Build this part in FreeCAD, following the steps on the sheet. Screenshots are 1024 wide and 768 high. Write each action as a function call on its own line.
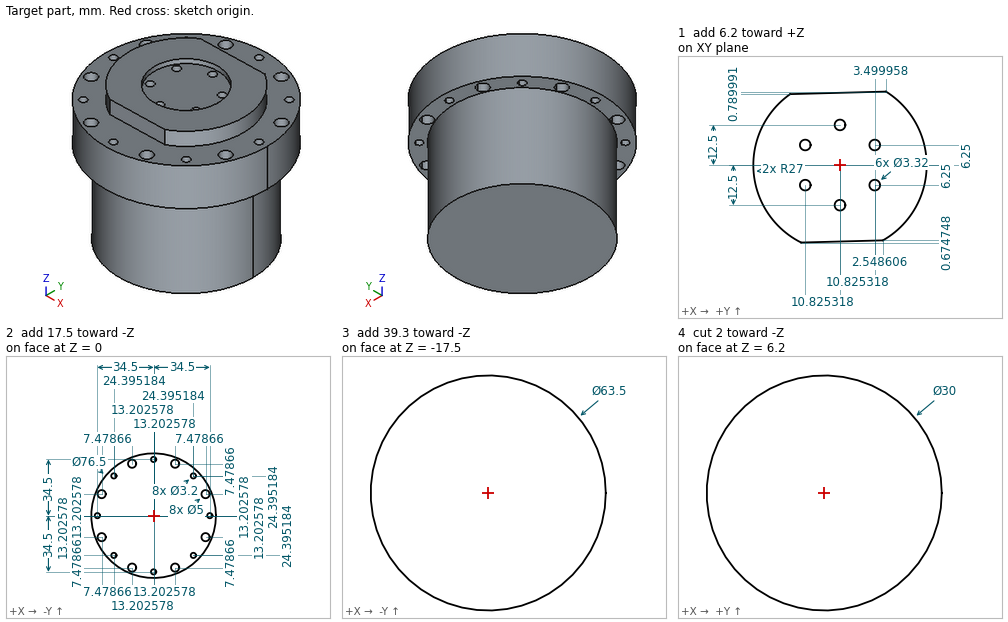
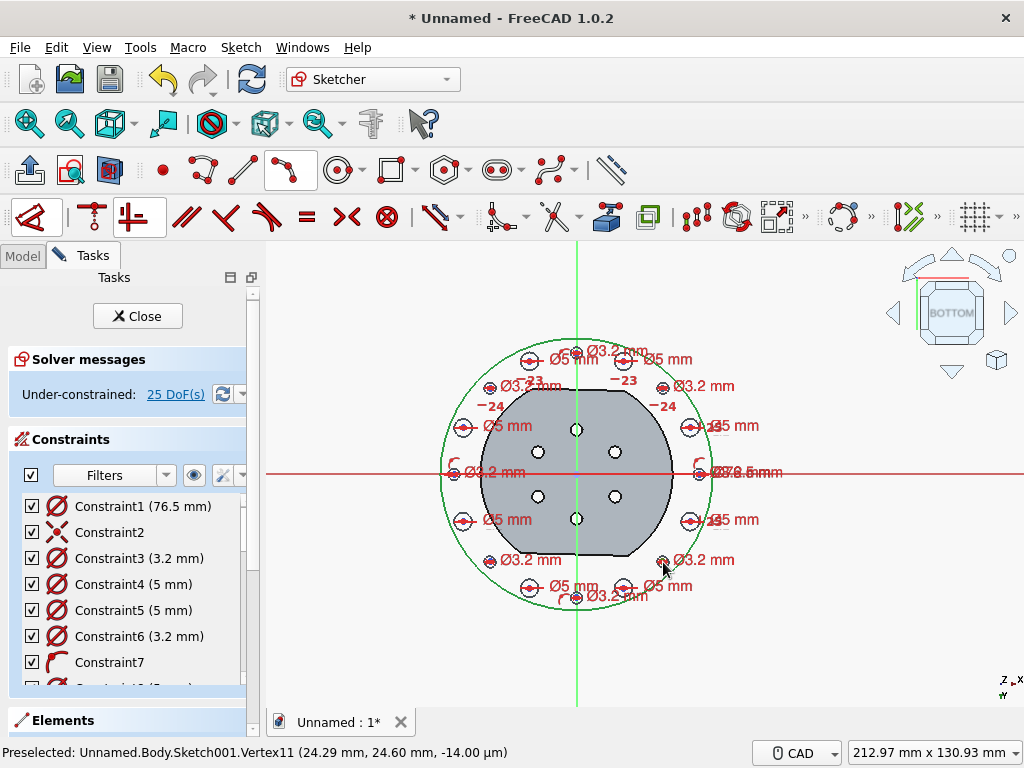
click(160, 218)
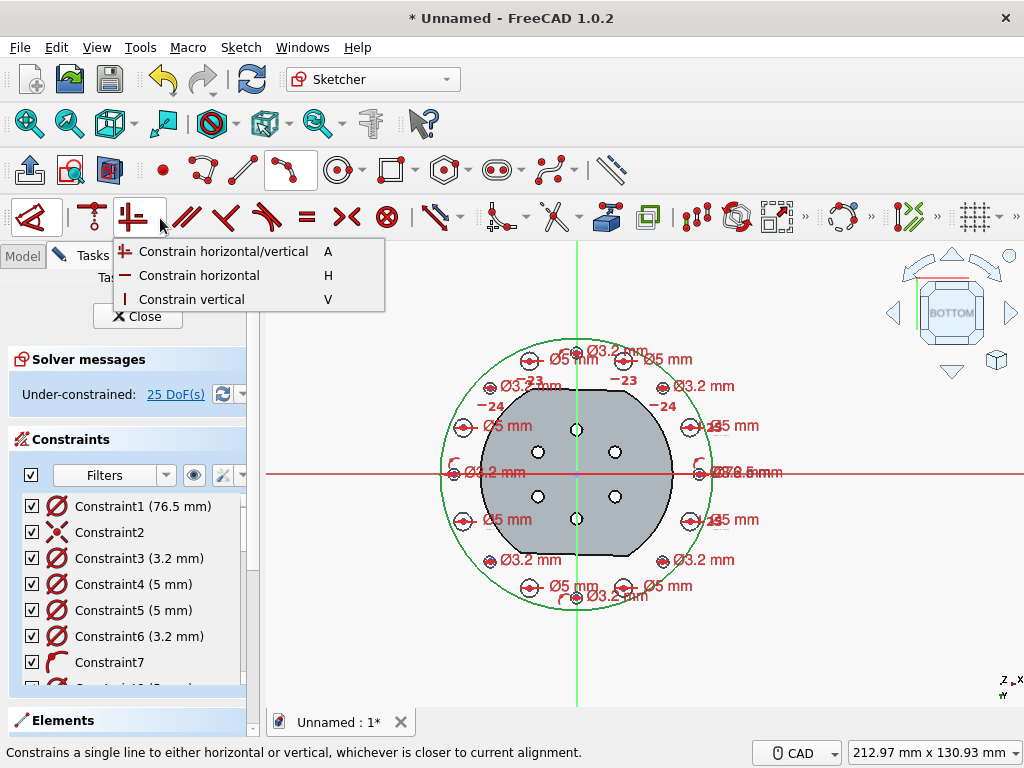
click(249, 299)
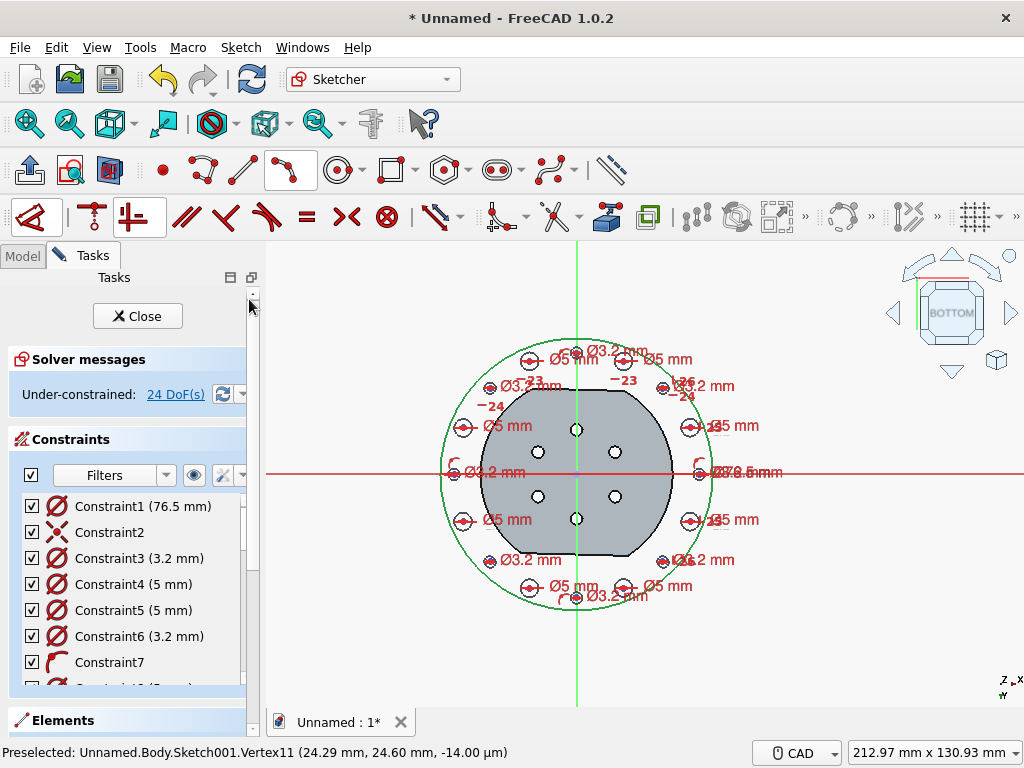
click(463, 428)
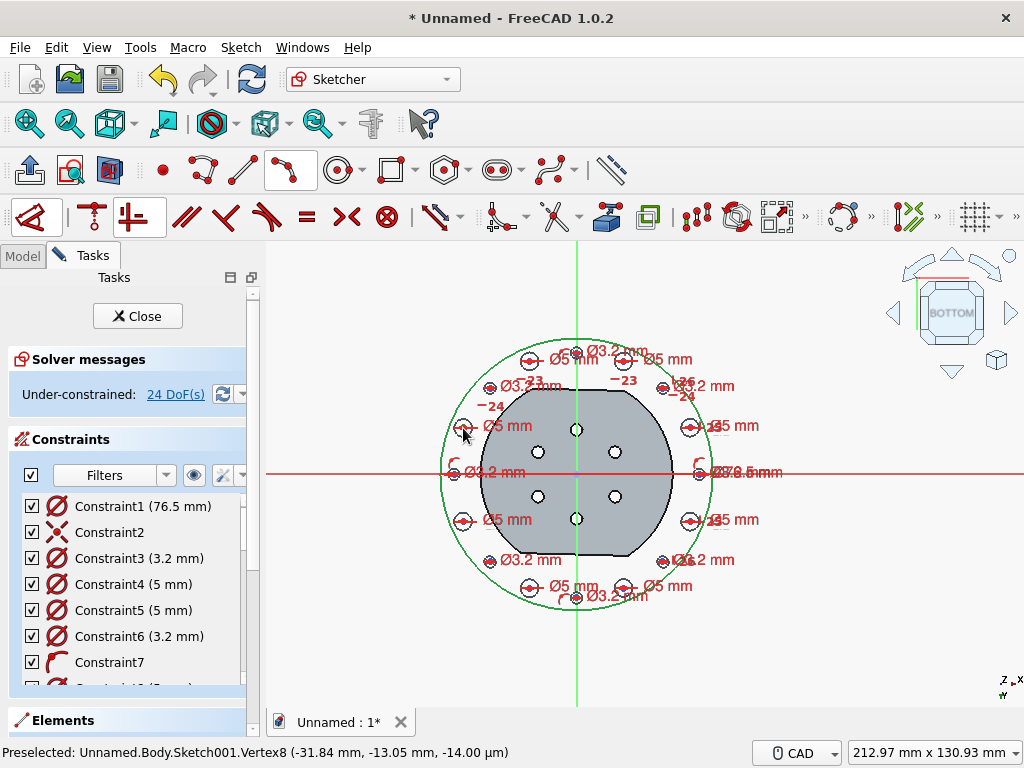
click(463, 522)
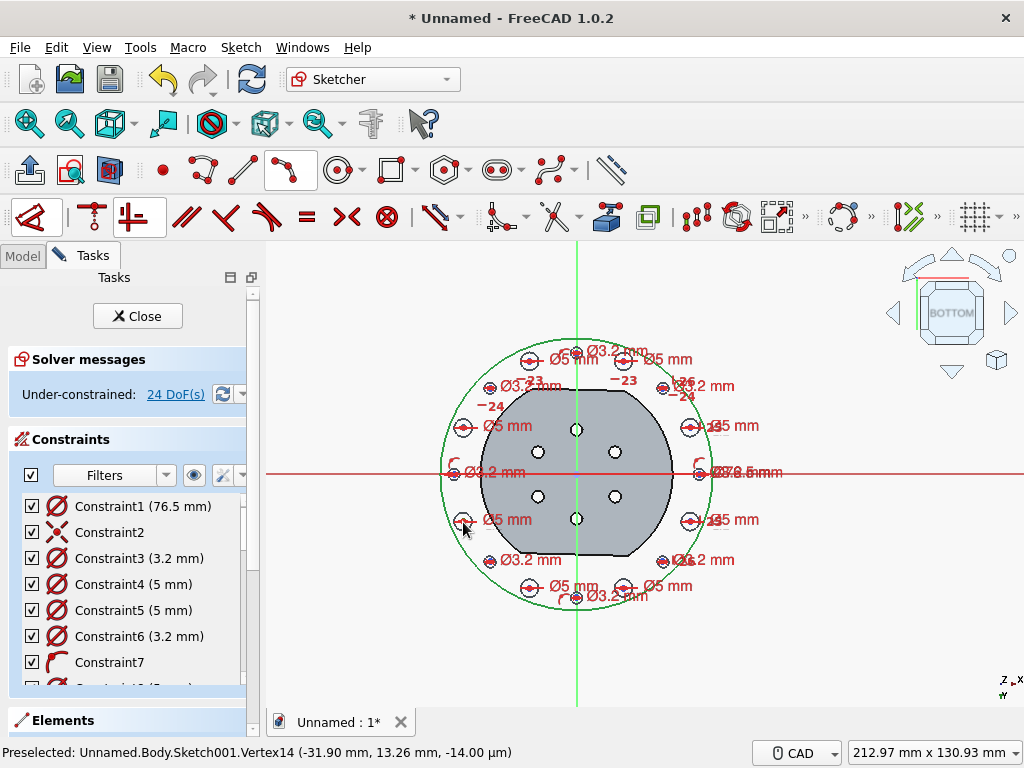
click(160, 218)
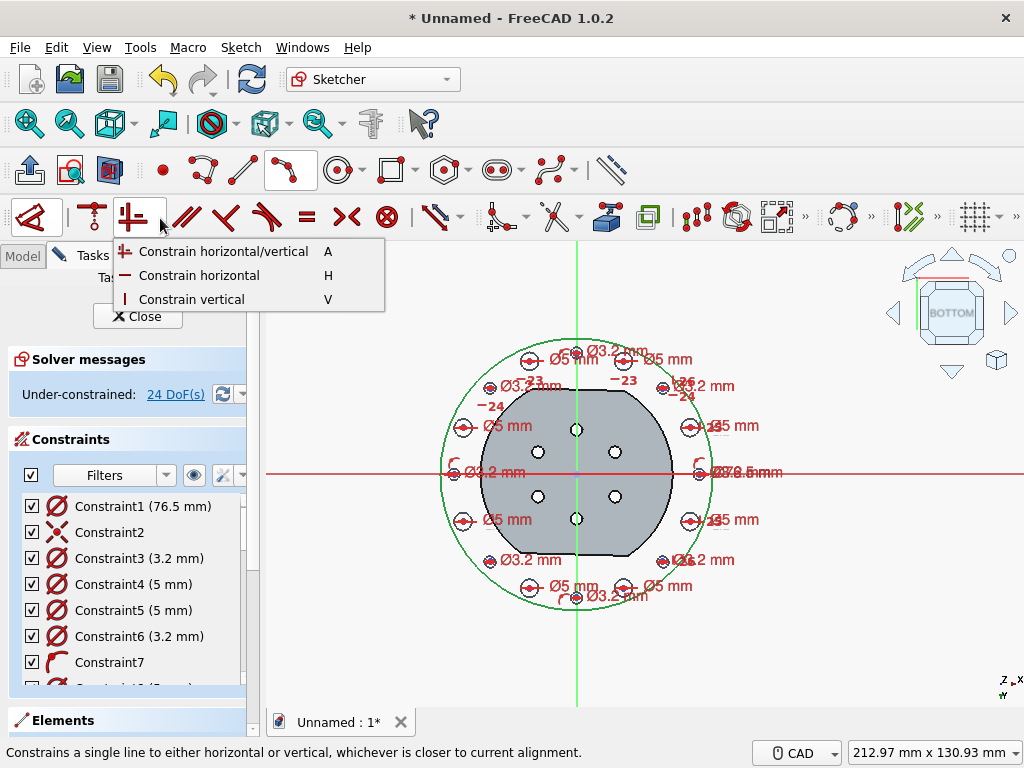
click(249, 299)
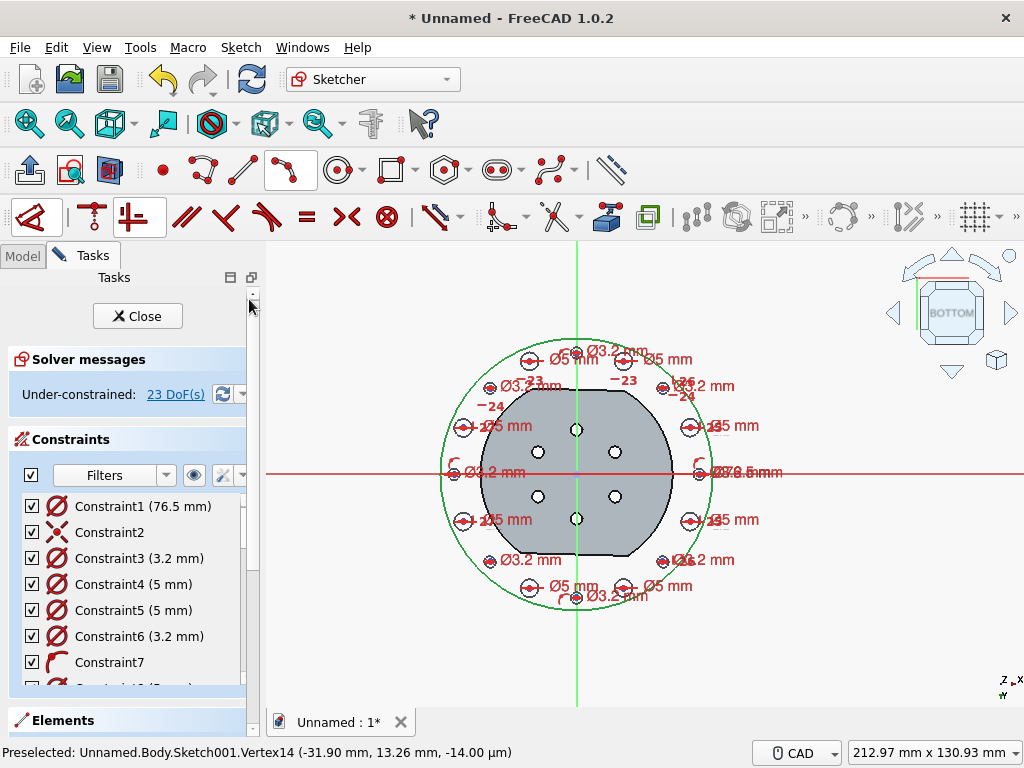
click(624, 588)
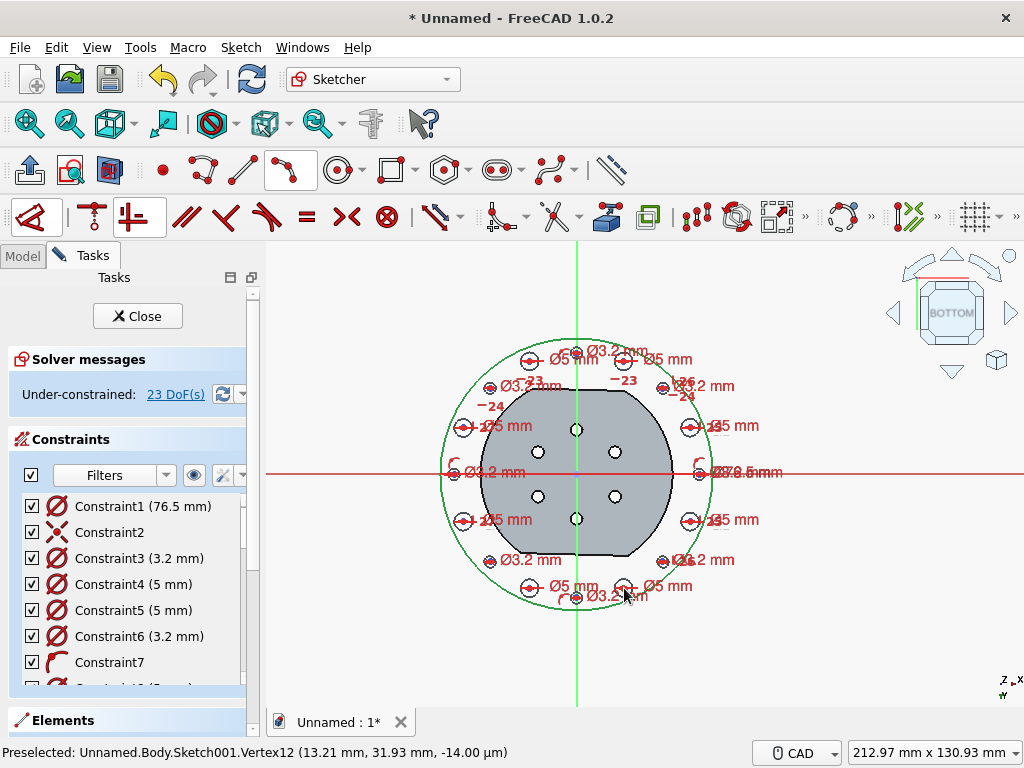
click(530, 588)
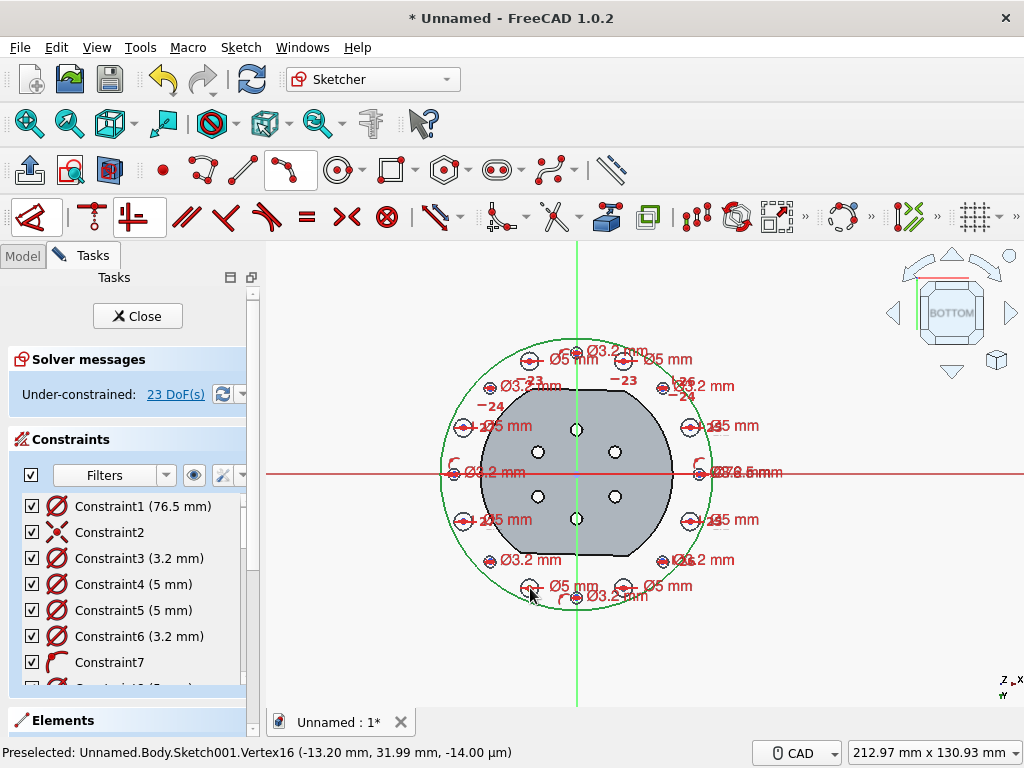
click(160, 218)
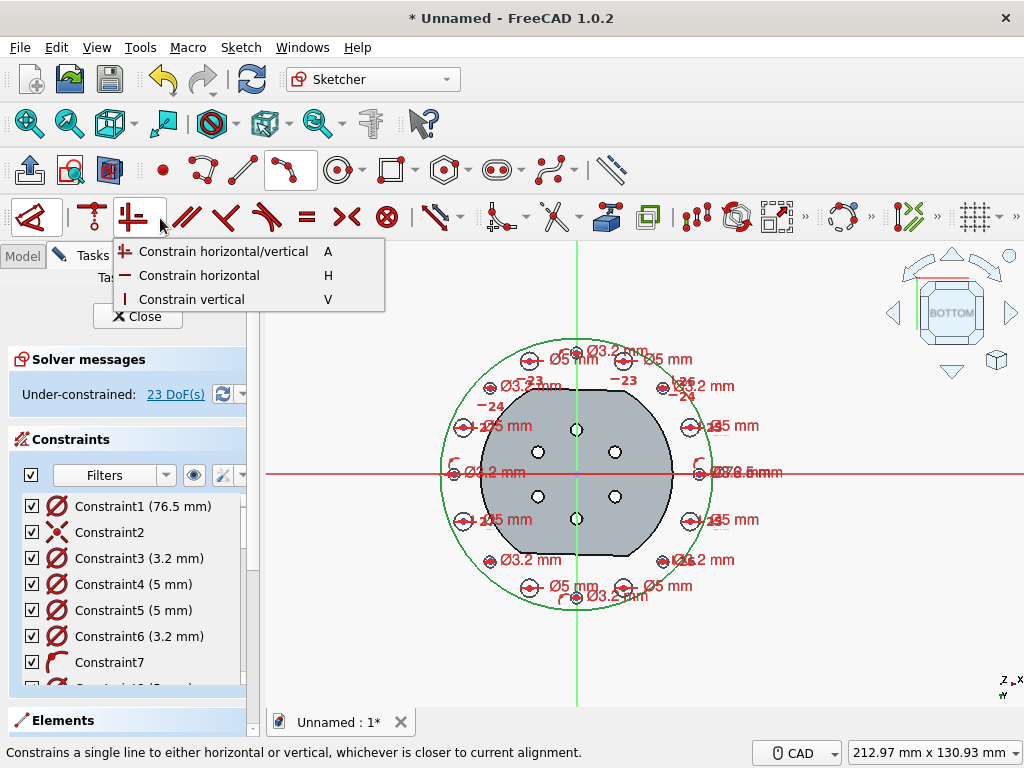
click(249, 275)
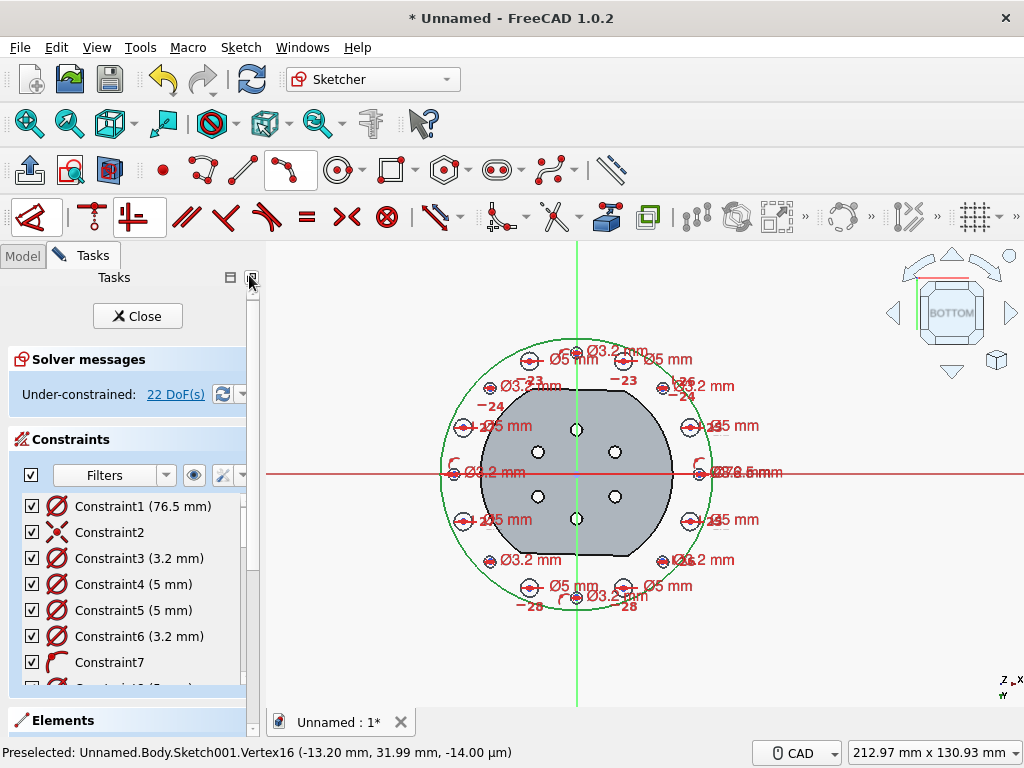
click(577, 353)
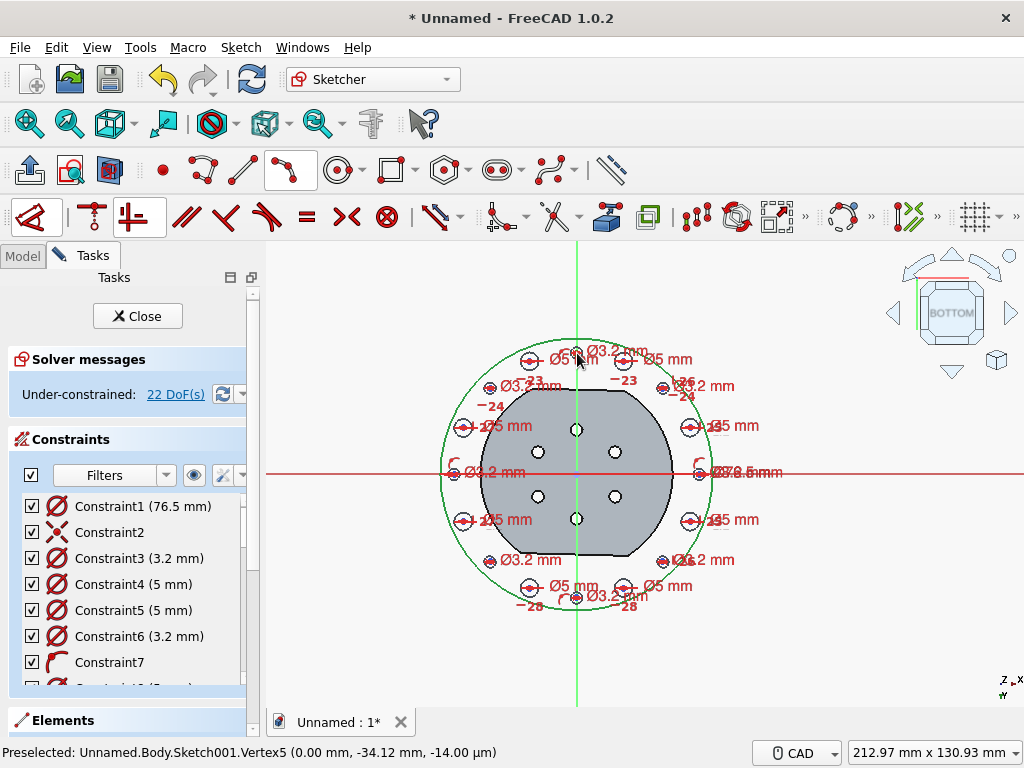
click(56, 218)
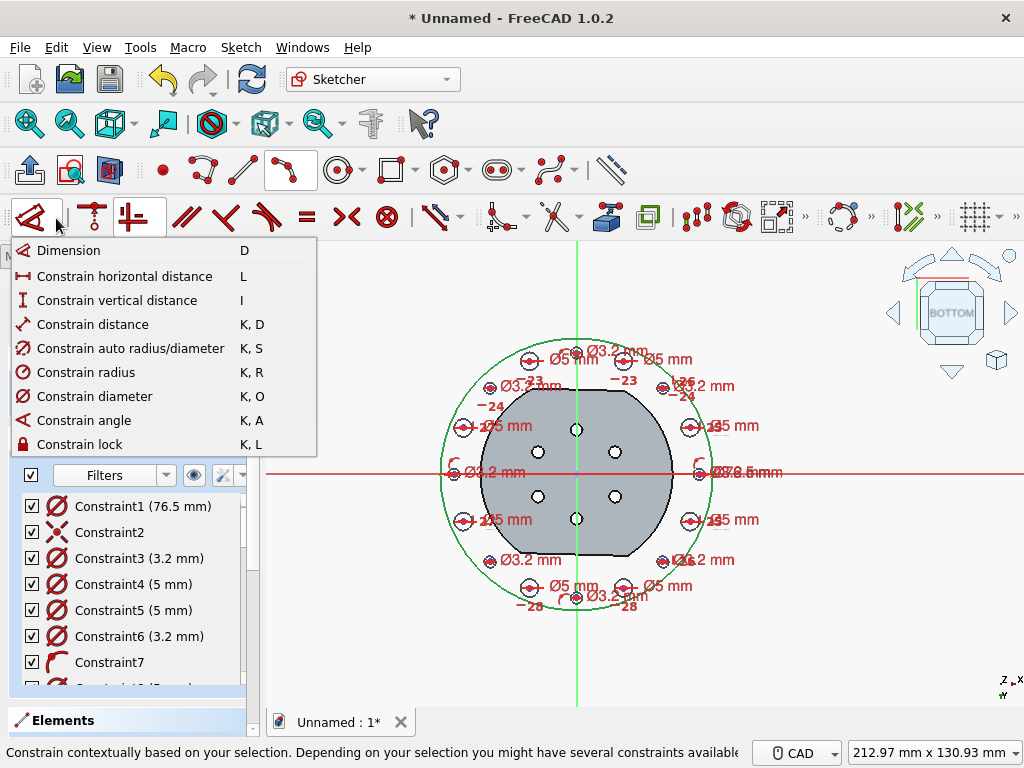
click(164, 300)